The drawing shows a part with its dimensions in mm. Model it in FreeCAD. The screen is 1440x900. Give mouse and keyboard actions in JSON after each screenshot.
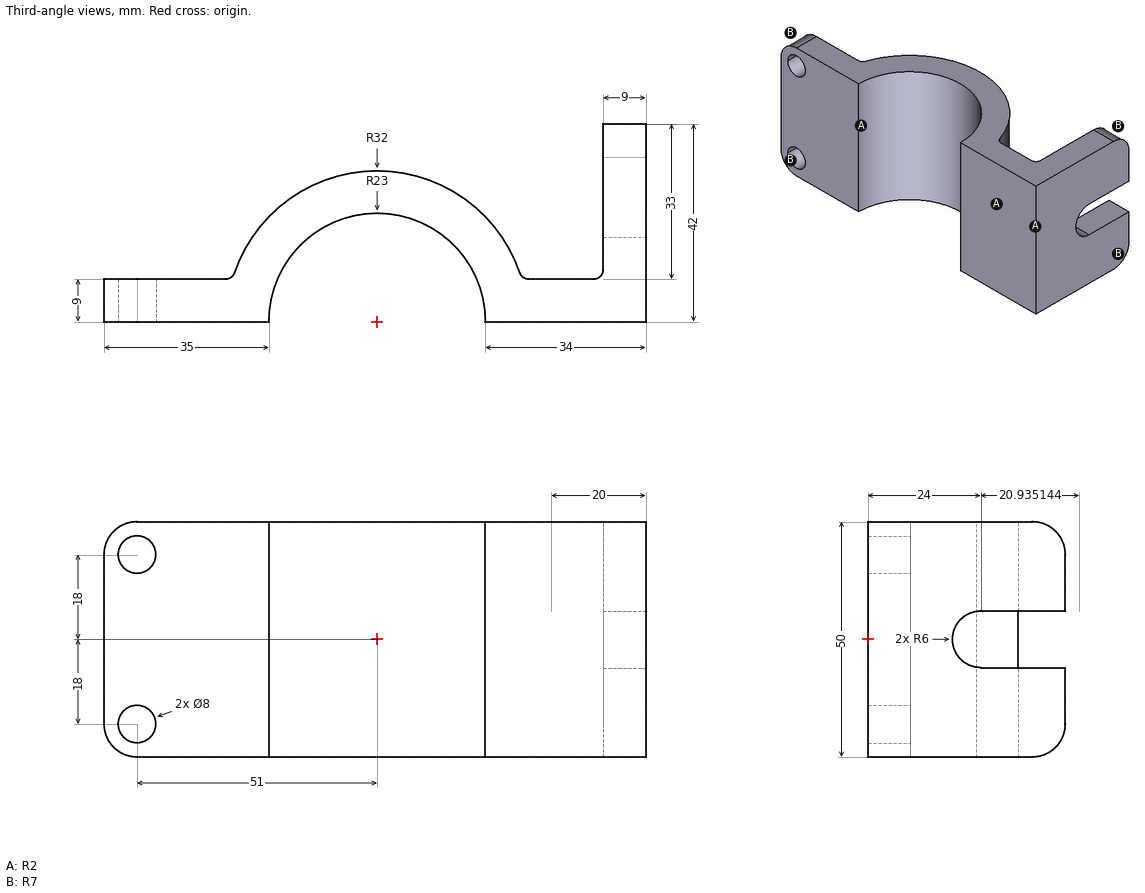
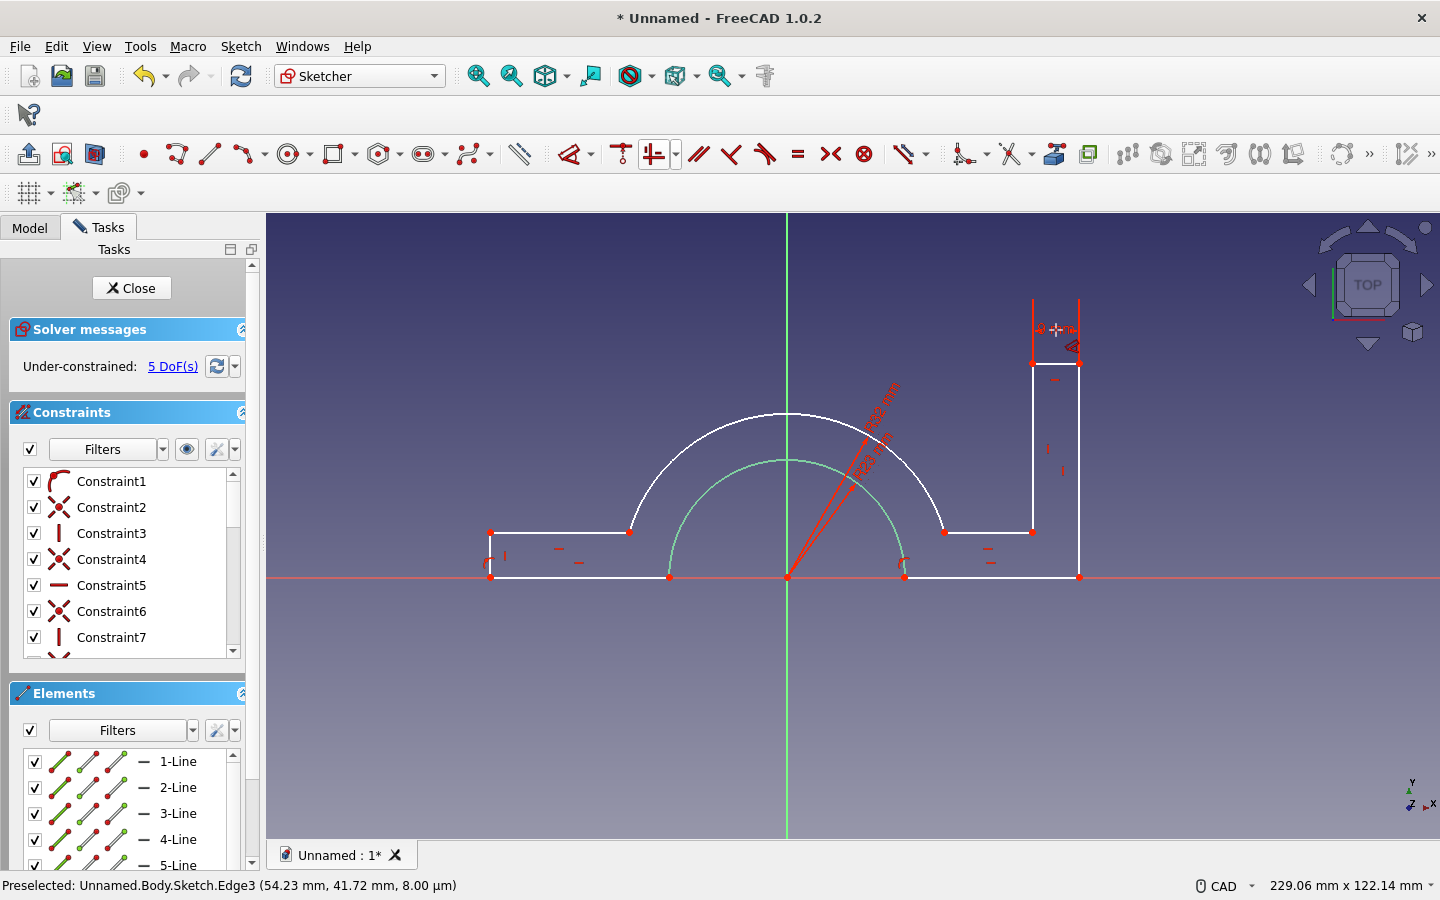
{"action": "left_click", "coordinate": [490, 546]}
{"action": "left_click", "coordinate": [456, 555]}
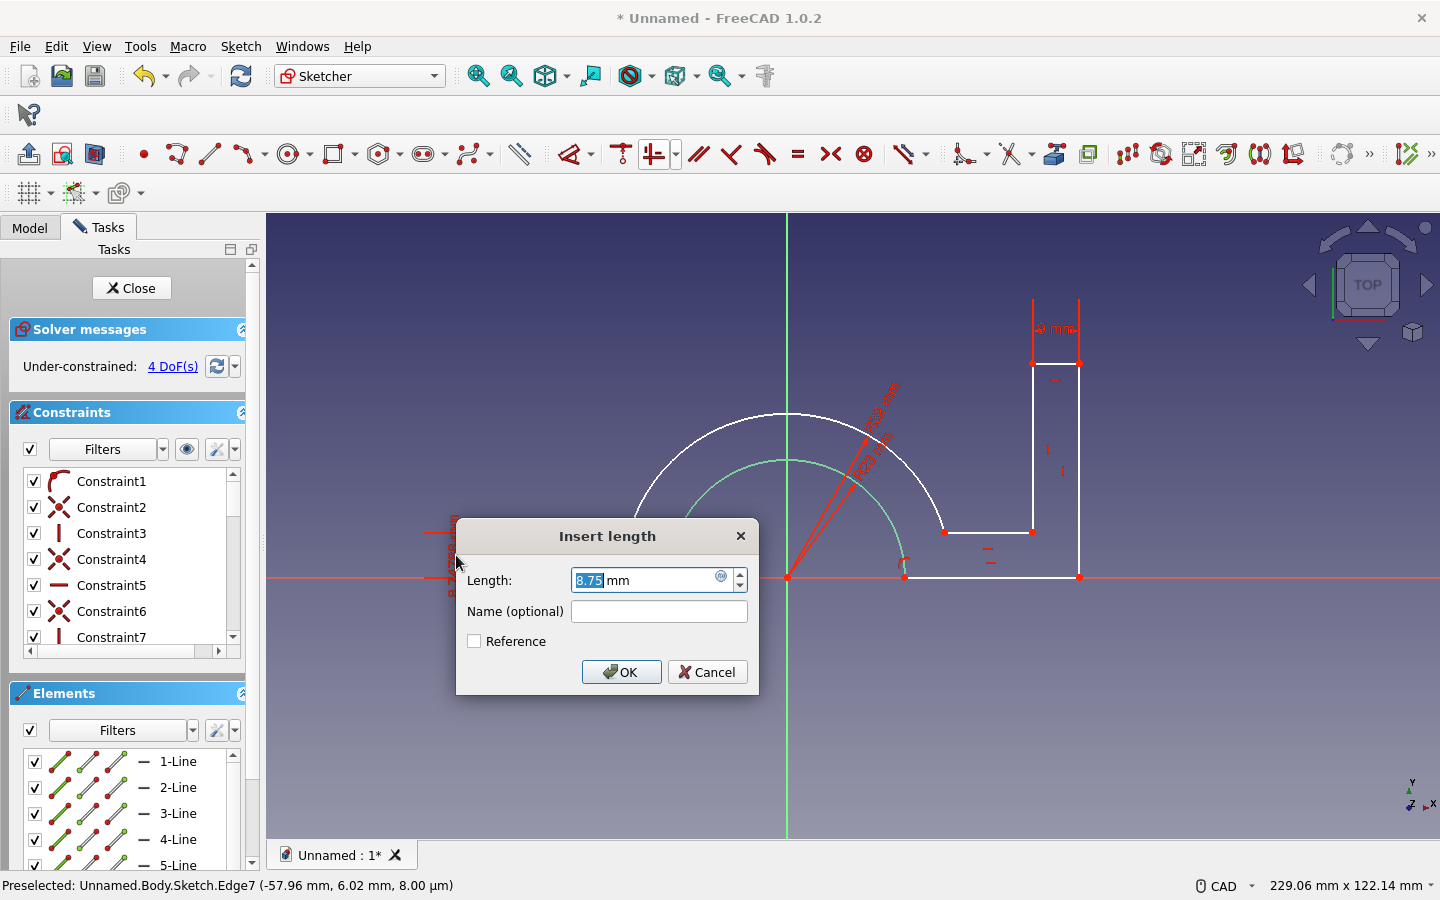
{"action": "type", "text": "9"}
{"action": "key", "text": "Return"}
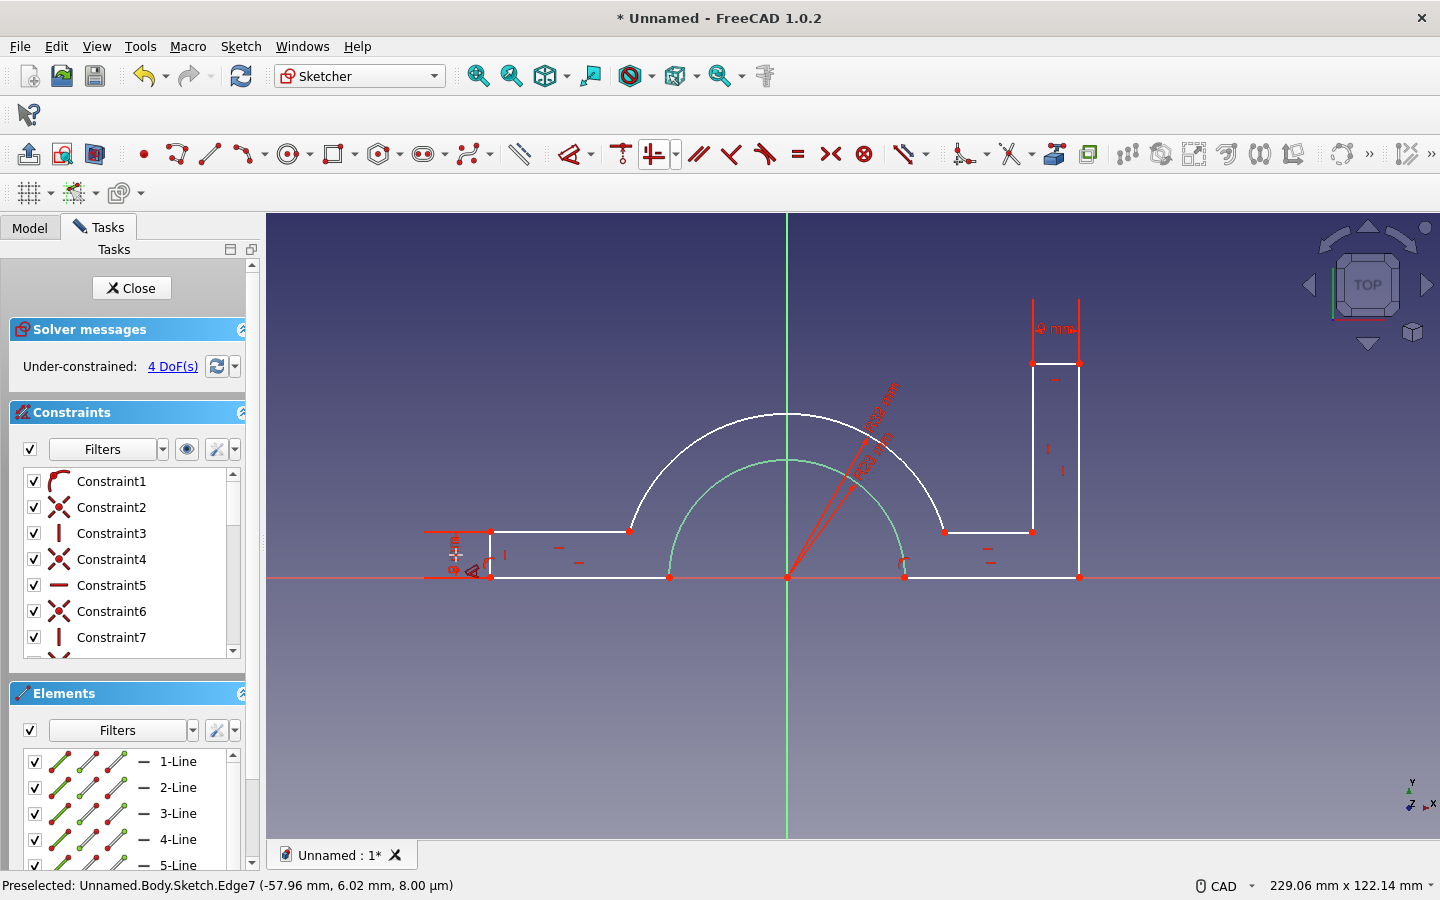
{"action": "left_click", "coordinate": [957, 578]}
{"action": "left_click", "coordinate": [992, 612]}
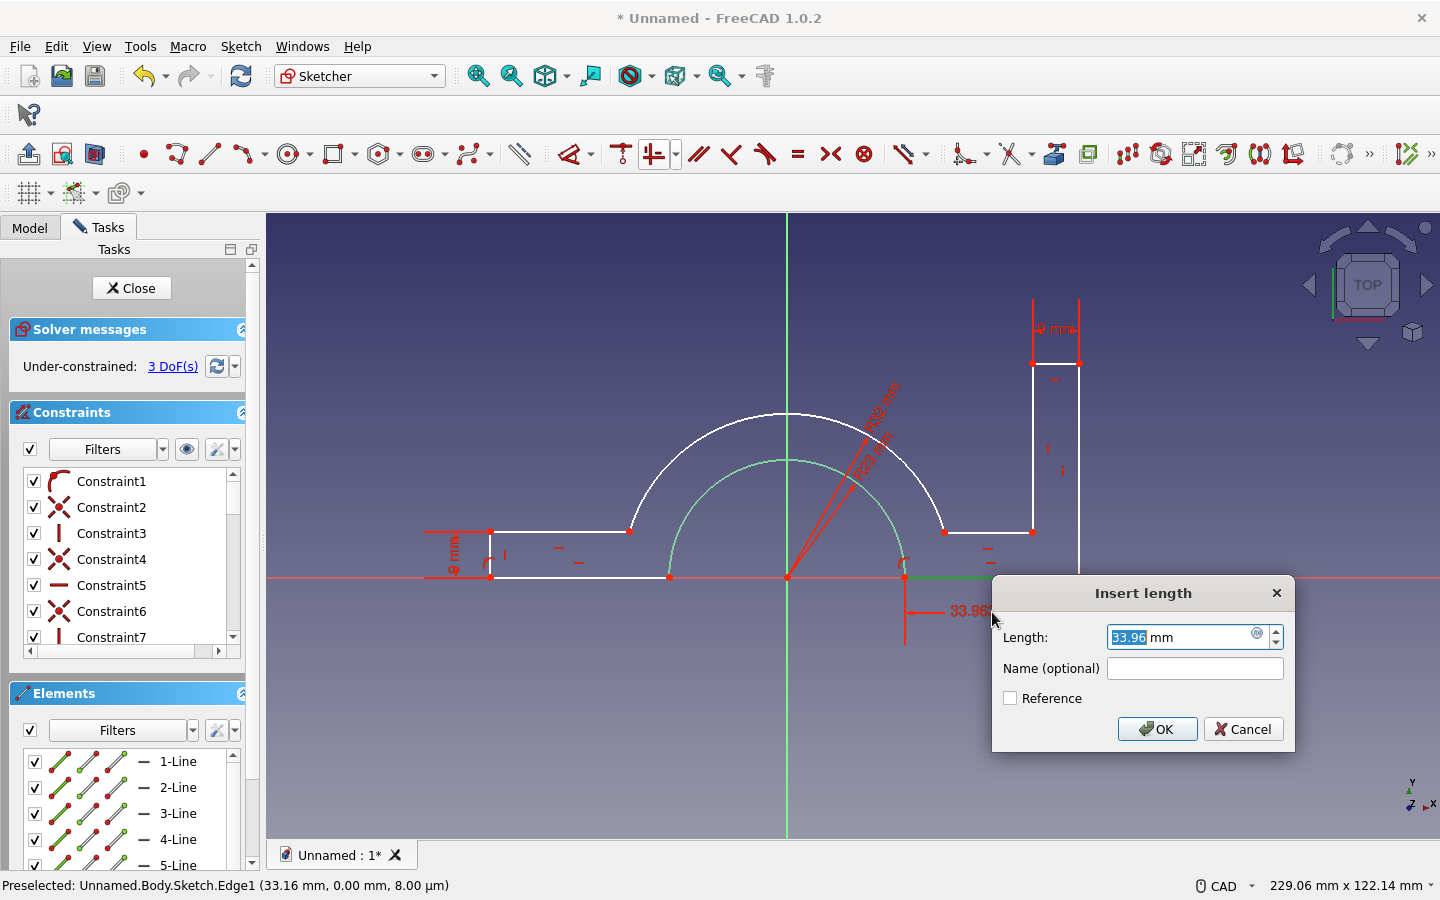
{"action": "type", "text": "34"}
{"action": "key", "text": "Return"}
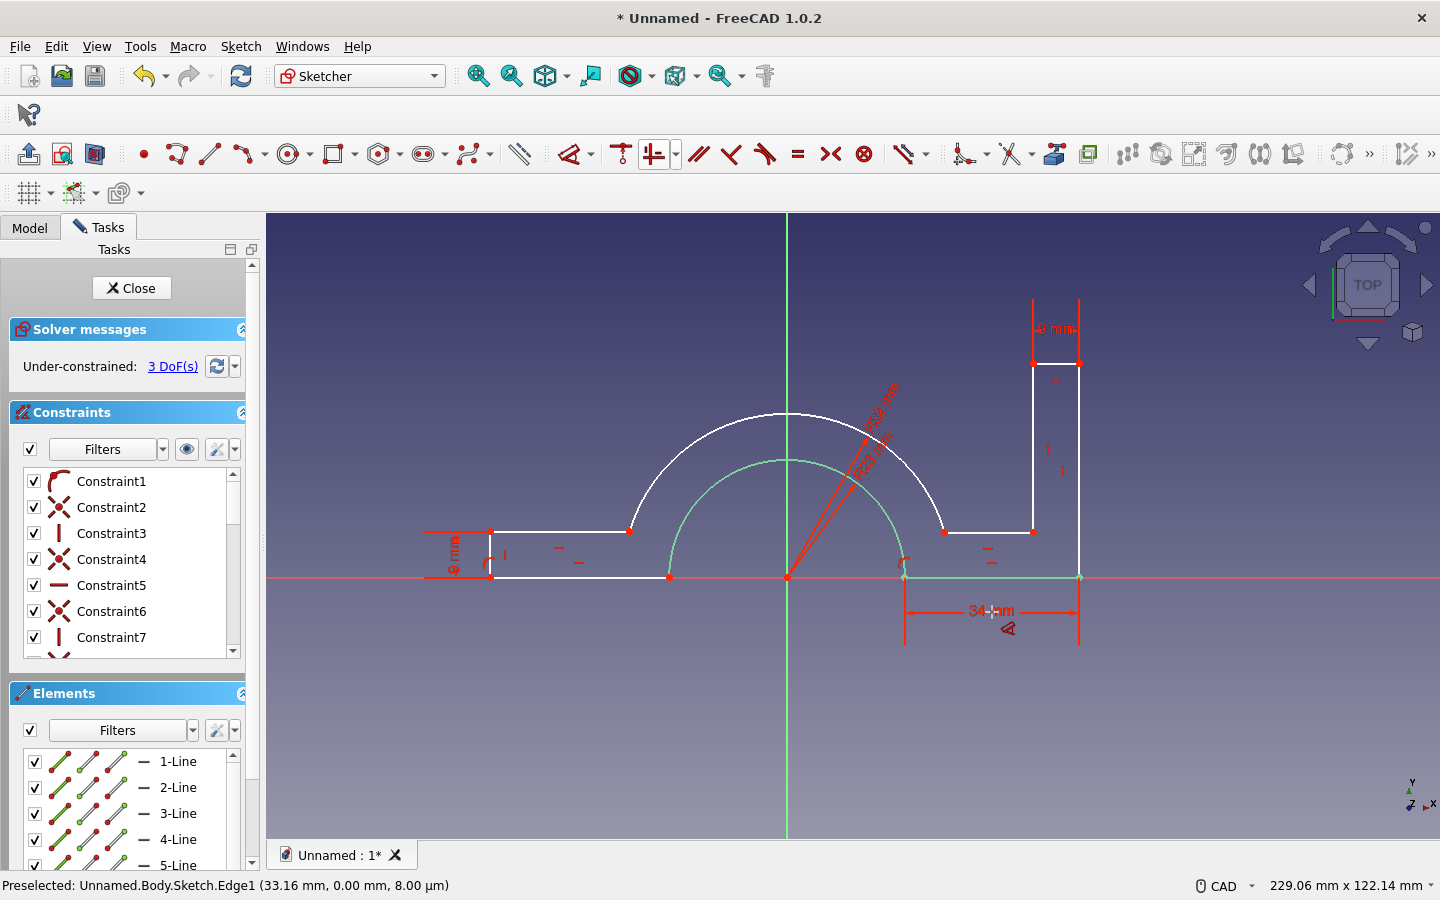
{"action": "left_click", "coordinate": [1079, 514]}
{"action": "left_click", "coordinate": [1113, 471]}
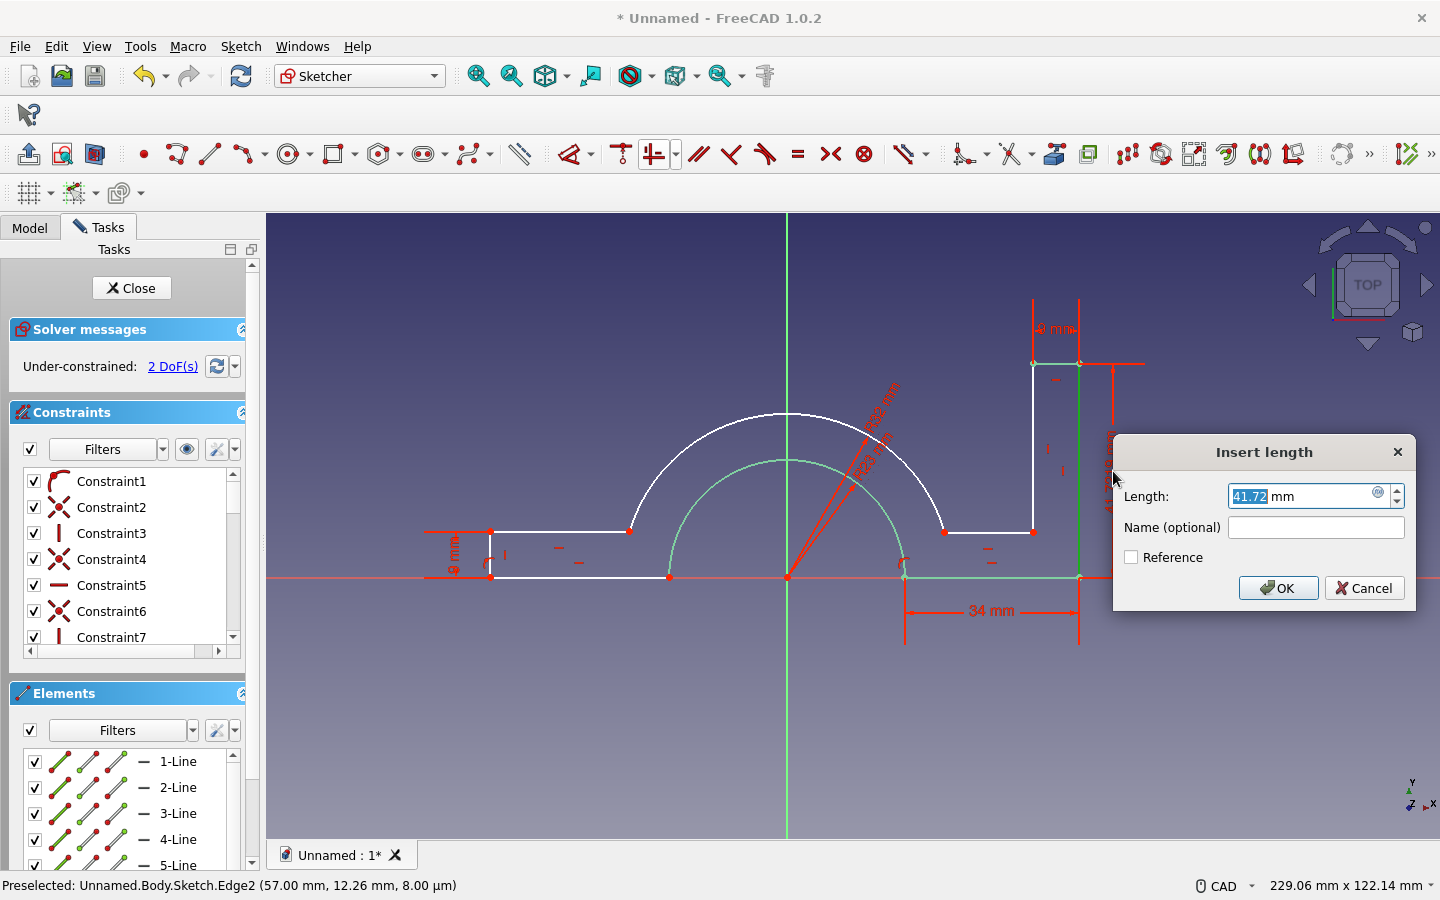
{"action": "type", "text": "42"}
{"action": "key", "text": "Return"}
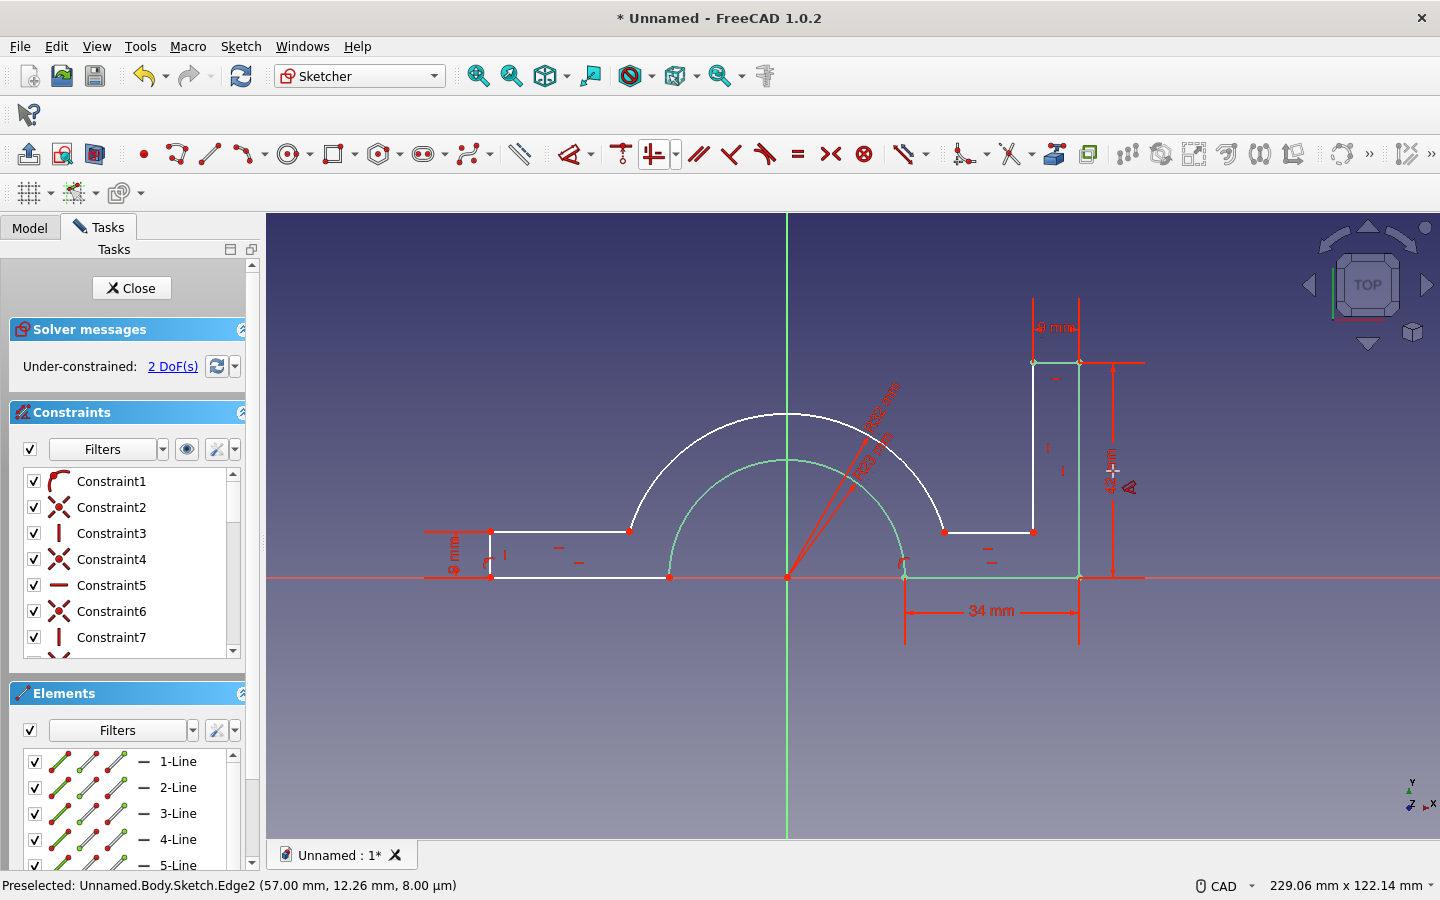
{"action": "left_click", "coordinate": [1033, 414]}
{"action": "left_click", "coordinate": [999, 448]}